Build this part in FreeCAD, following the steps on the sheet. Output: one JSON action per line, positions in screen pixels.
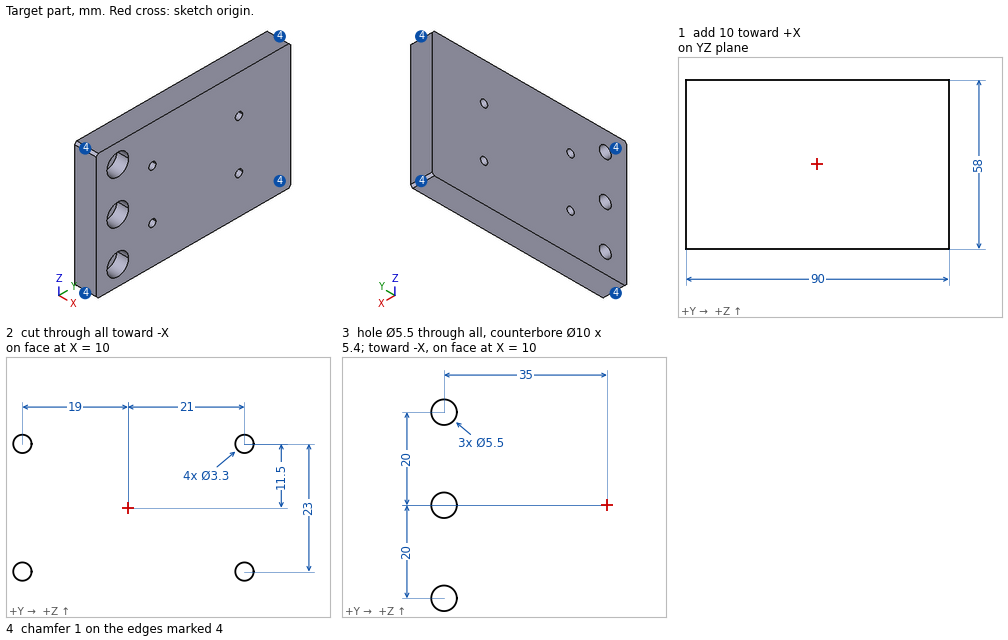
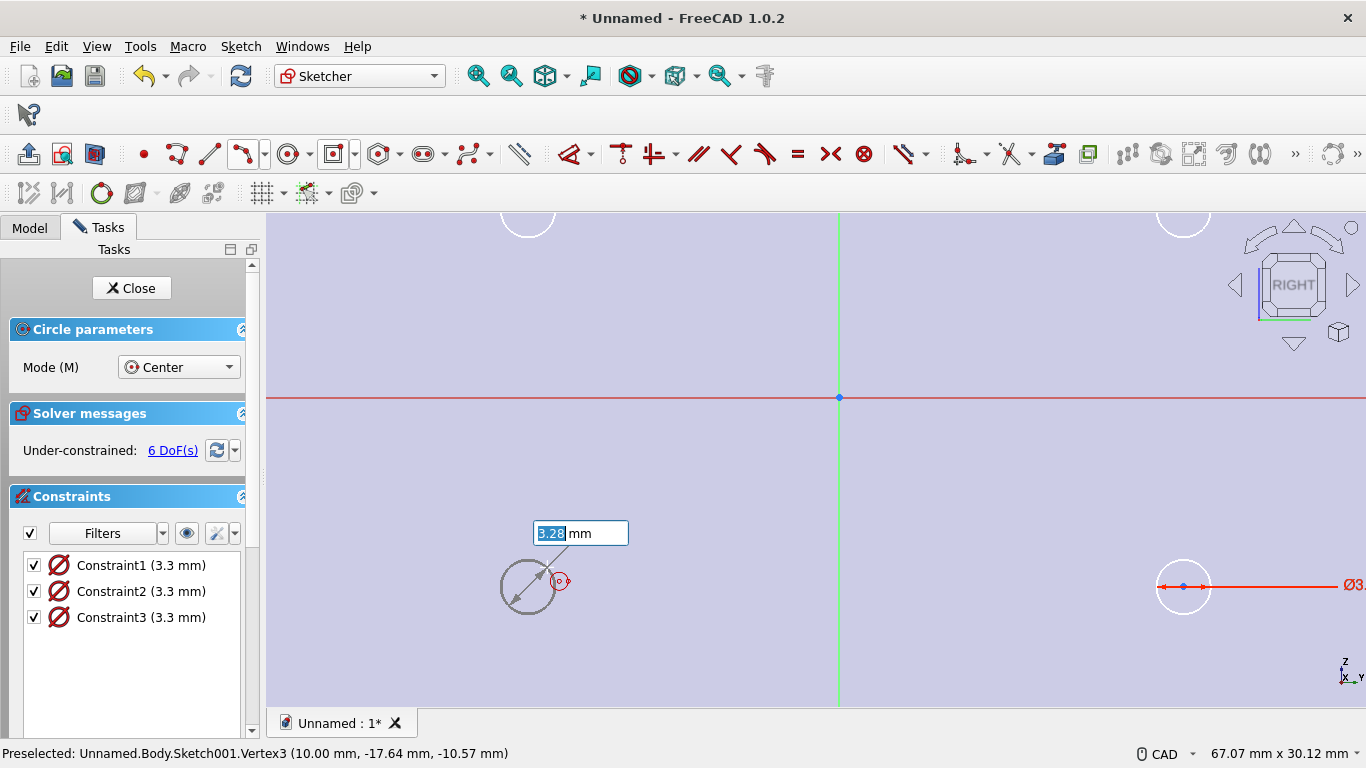
{"action": "type", "text": "3.3"}
{"action": "key", "text": "Return"}
{"action": "key", "text": "Escape"}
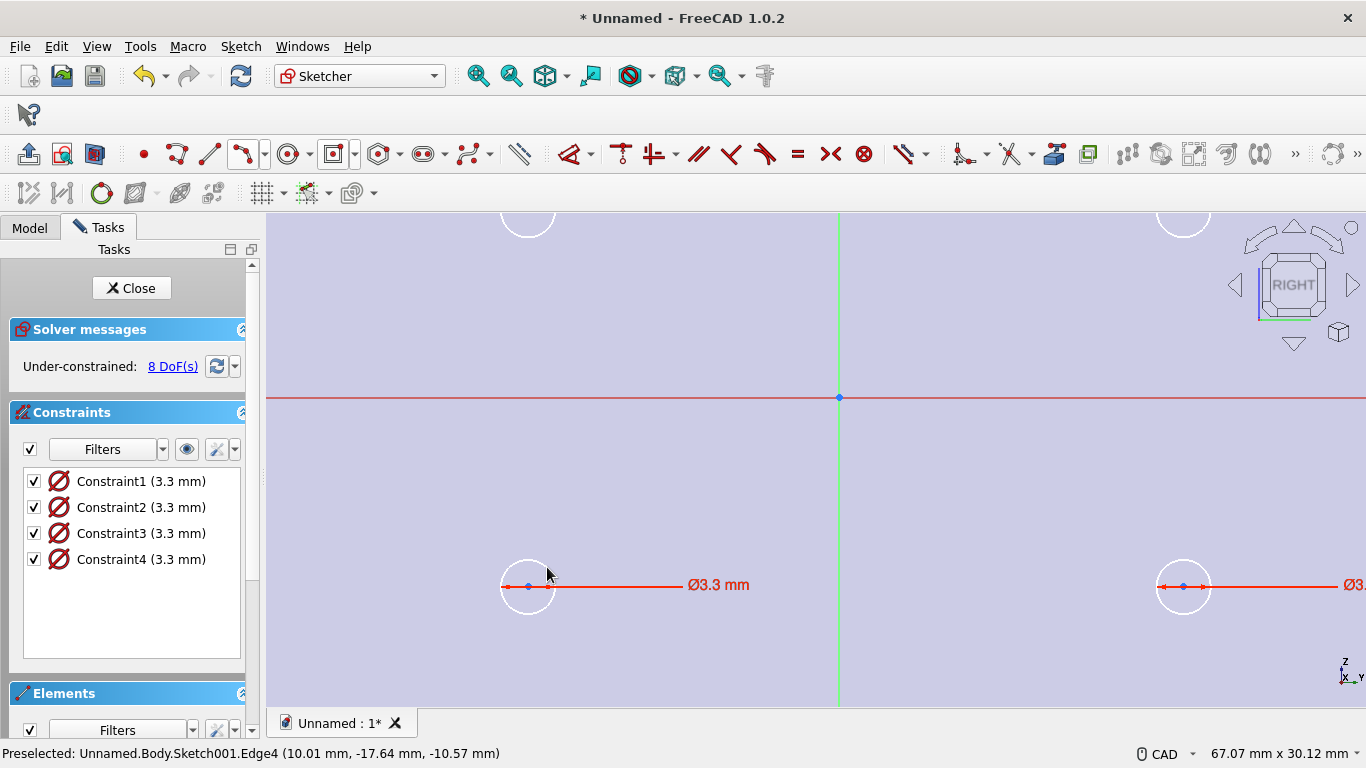
{"action": "scroll", "coordinate": [528, 587], "scroll_direction": "down", "scroll_amount": 2}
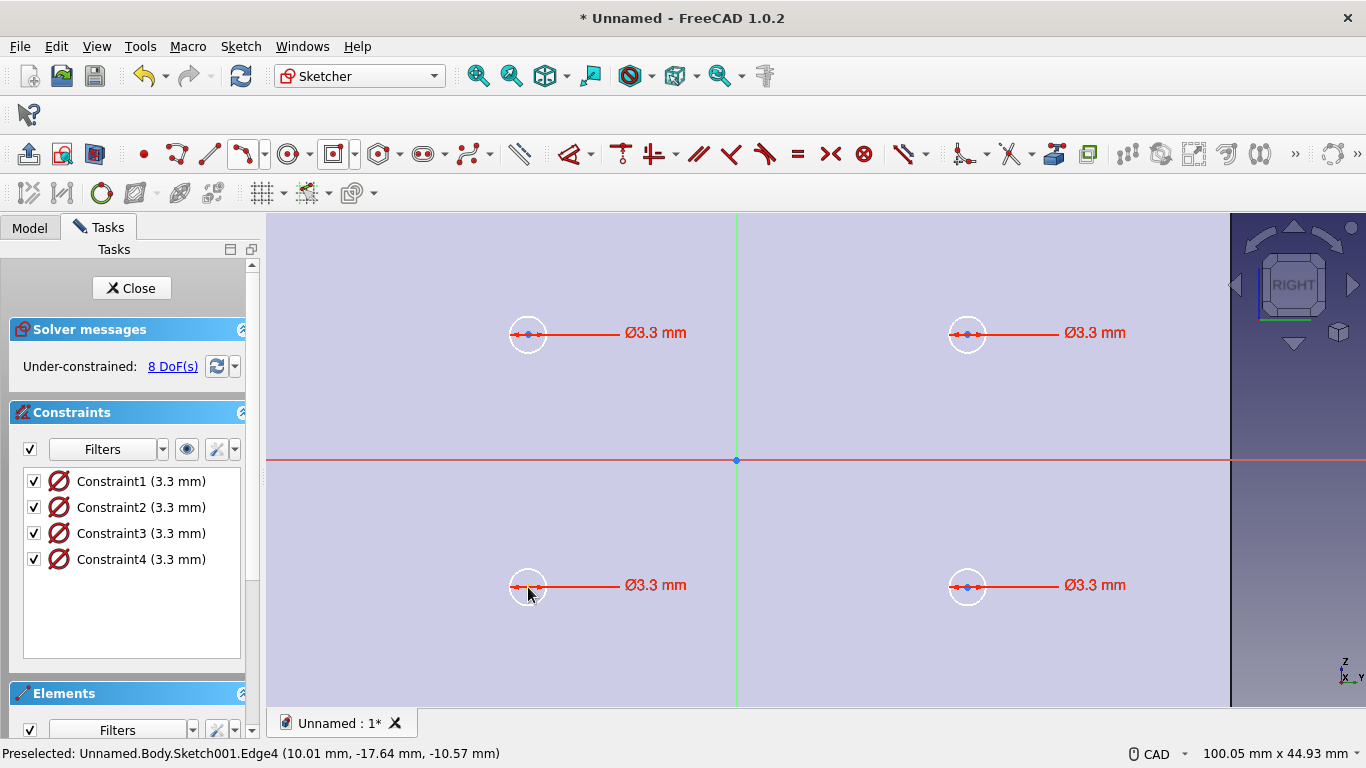
{"action": "left_click", "coordinate": [968, 335]}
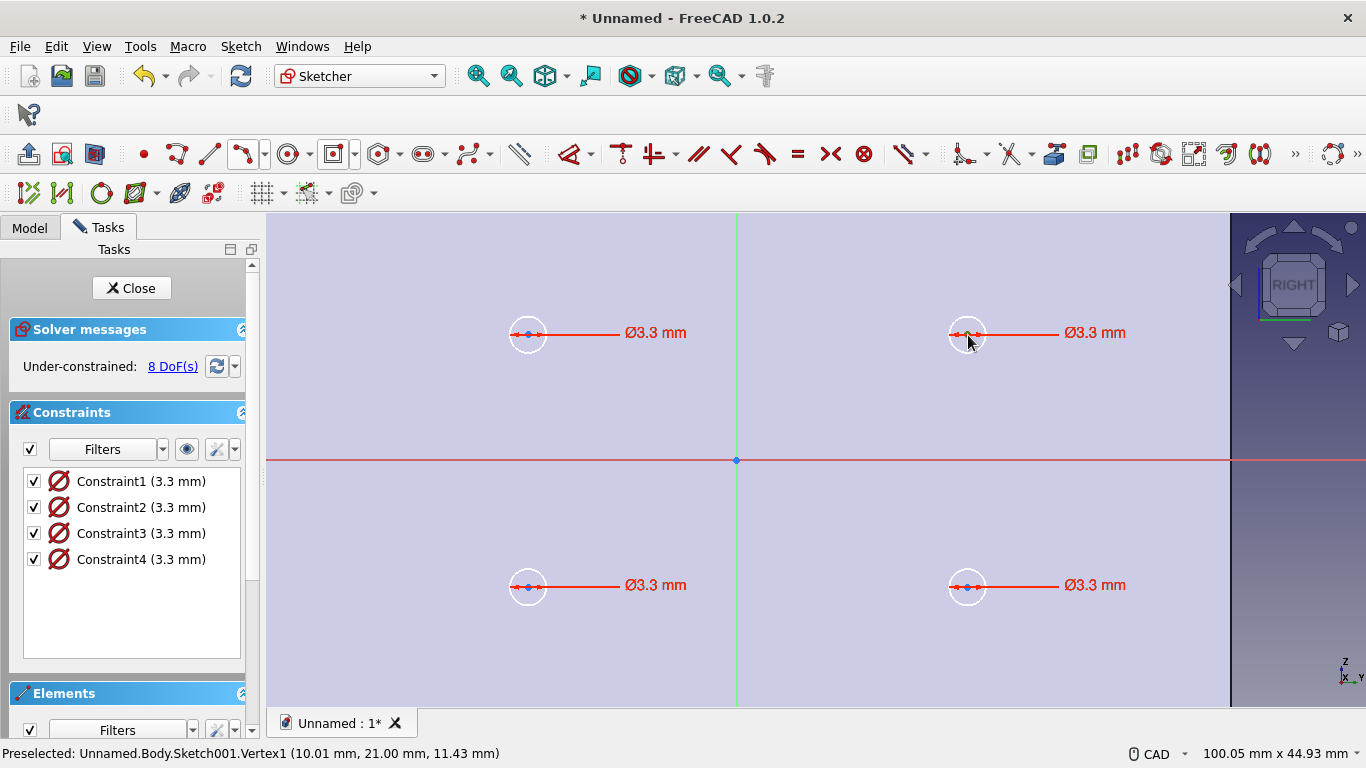
{"action": "left_click", "coordinate": [968, 587]}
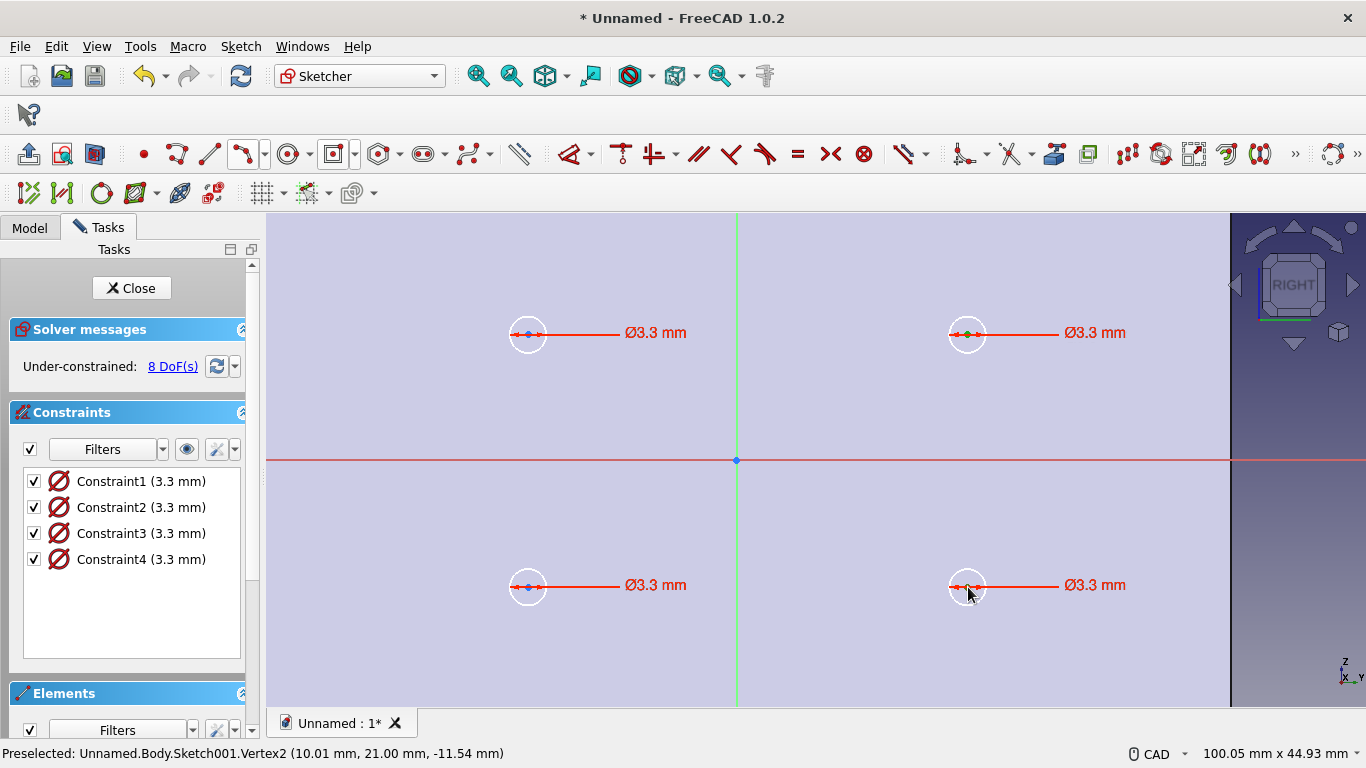
{"action": "left_click", "coordinate": [676, 154]}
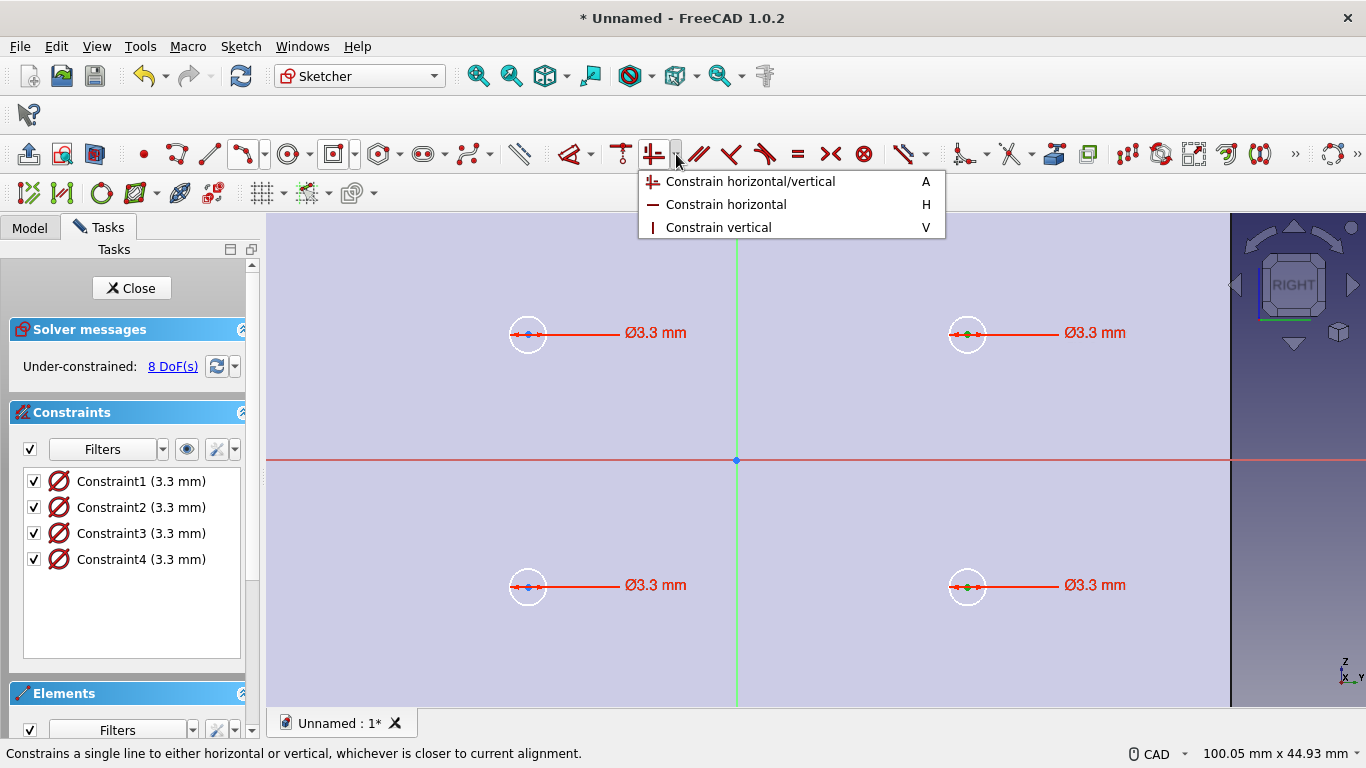
{"action": "left_click", "coordinate": [792, 228]}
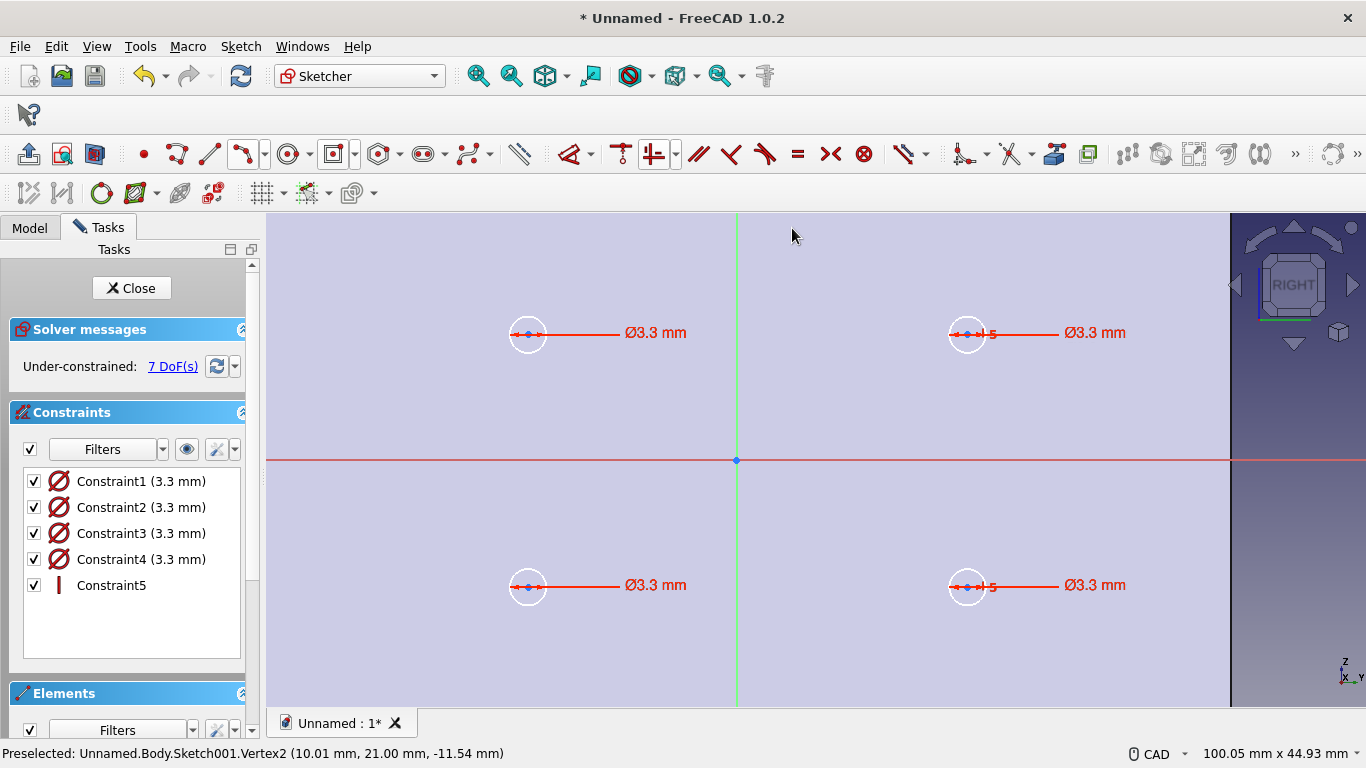
{"action": "left_click", "coordinate": [968, 335]}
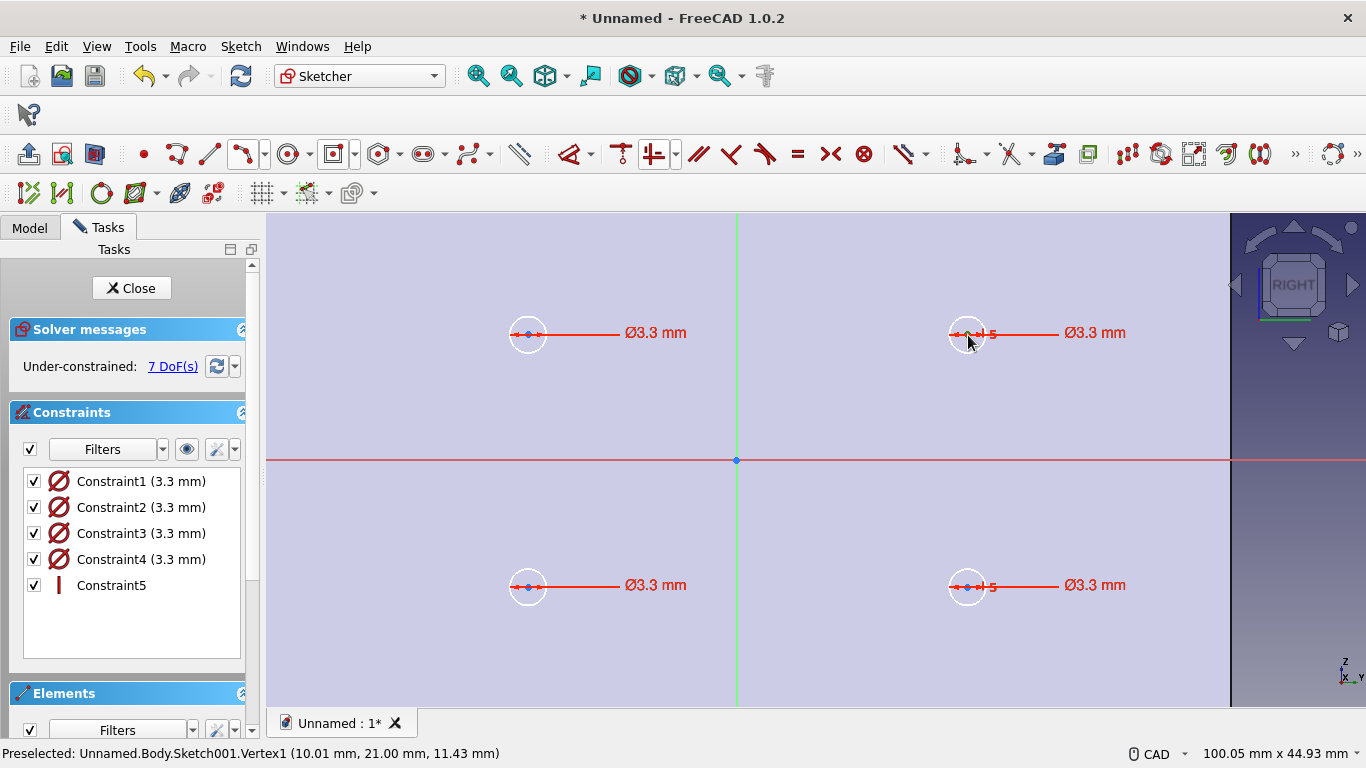
{"action": "left_click", "coordinate": [528, 335]}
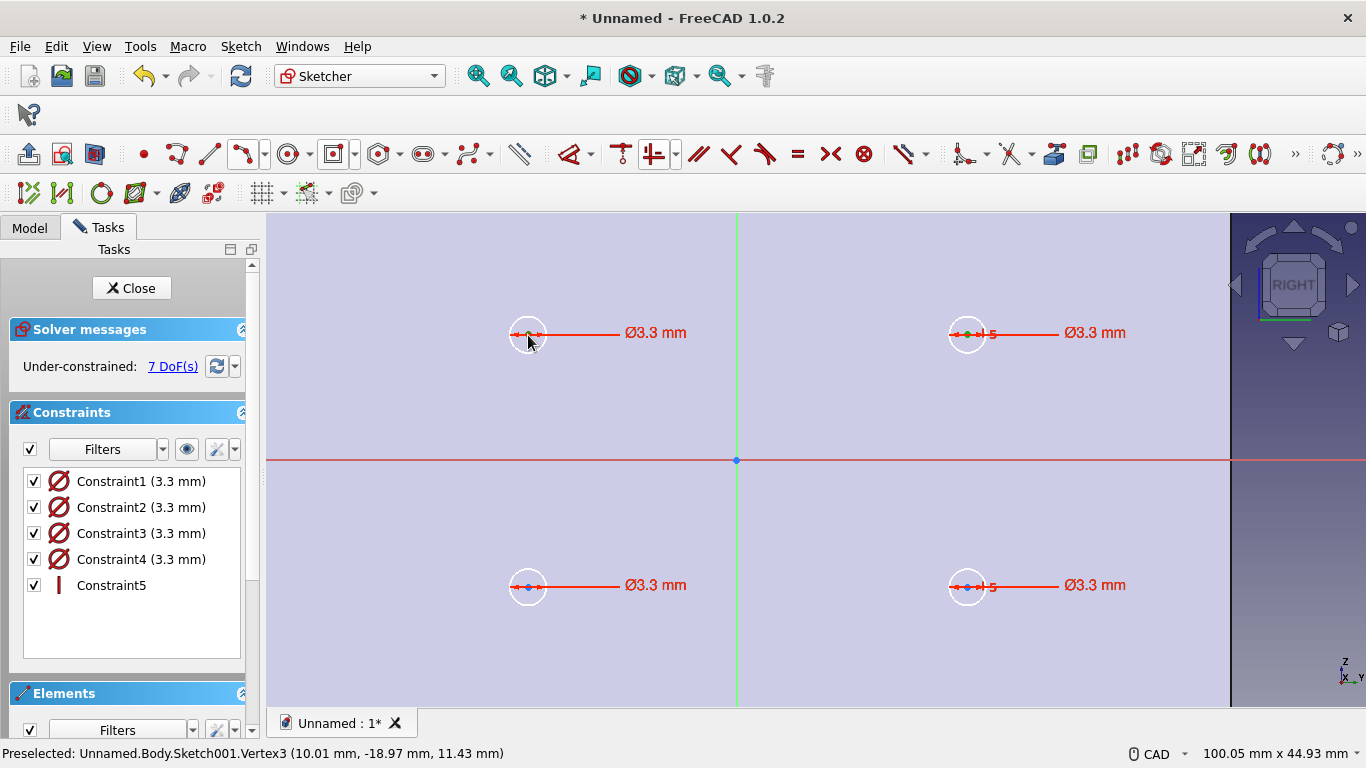
{"action": "left_click", "coordinate": [676, 154]}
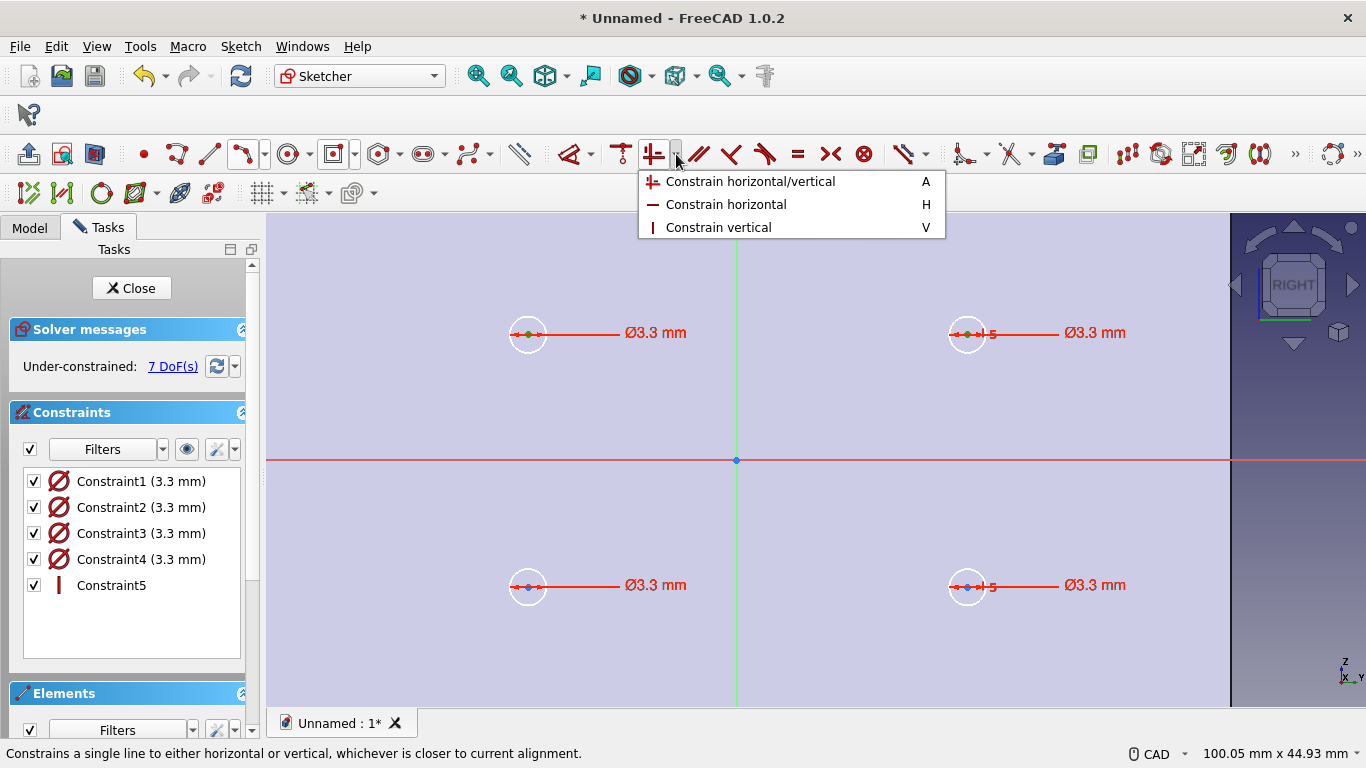
{"action": "left_click", "coordinate": [792, 204]}